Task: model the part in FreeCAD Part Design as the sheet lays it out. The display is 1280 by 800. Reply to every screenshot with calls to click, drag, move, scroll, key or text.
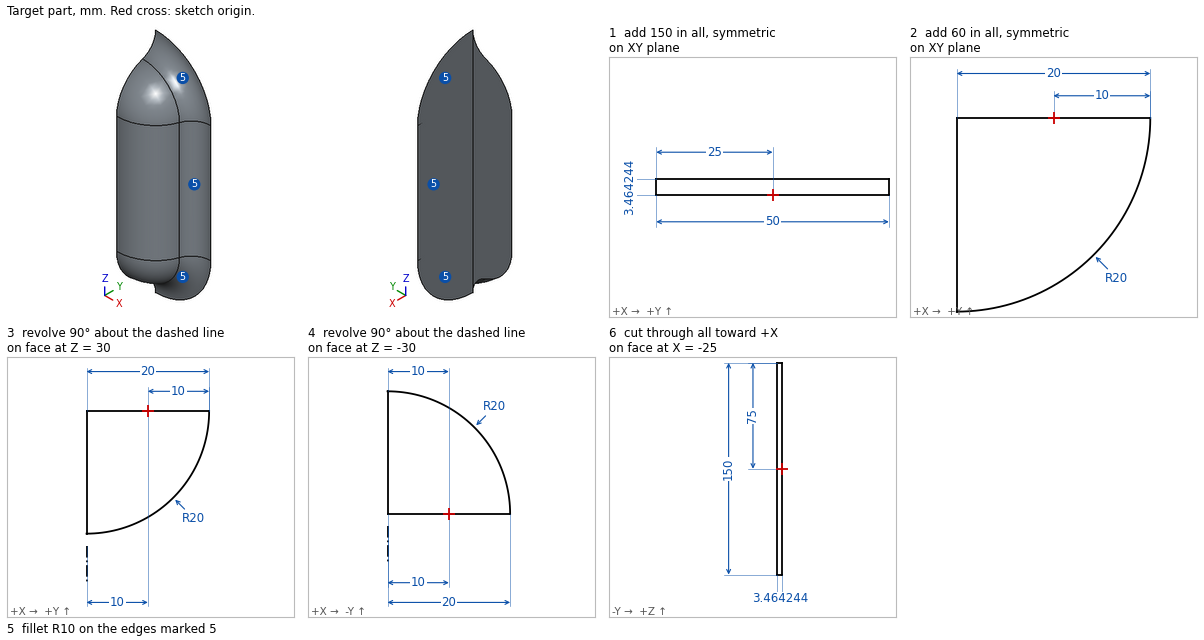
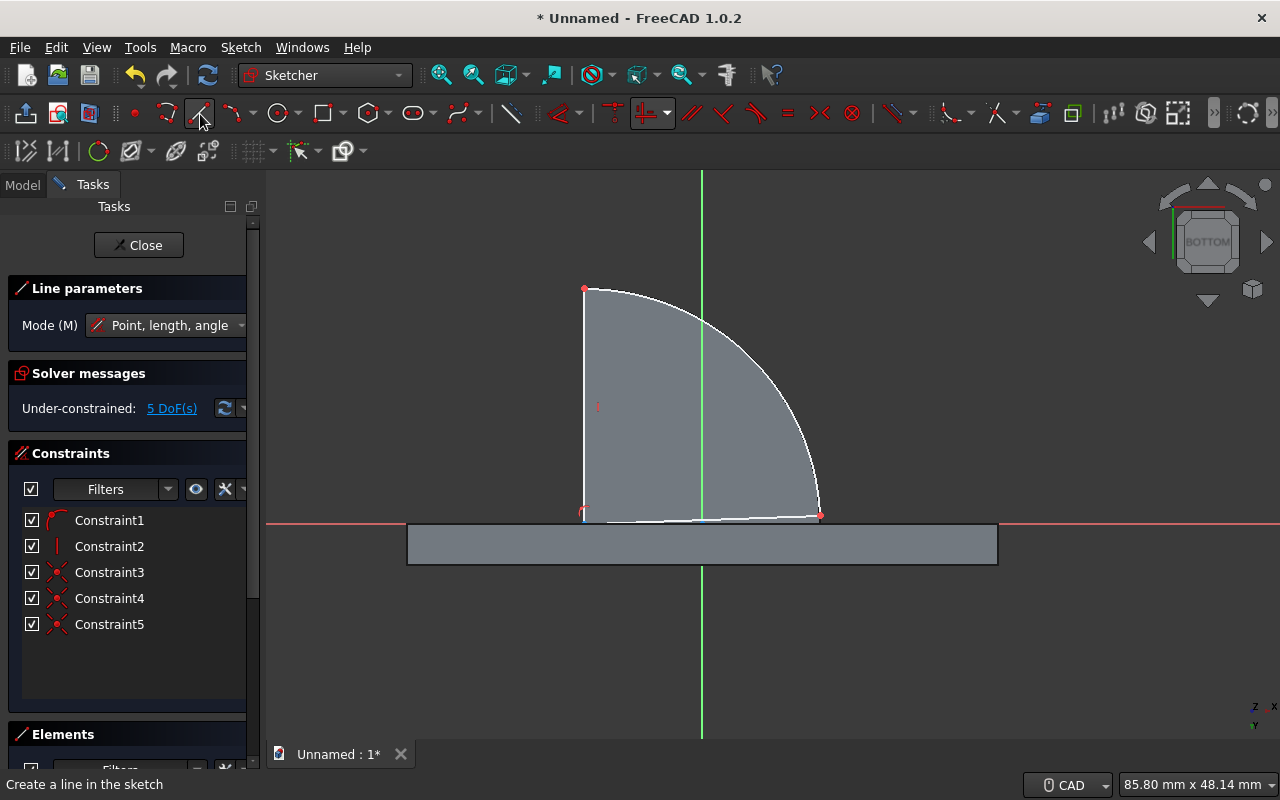
click(584, 548)
click(584, 619)
key(Escape)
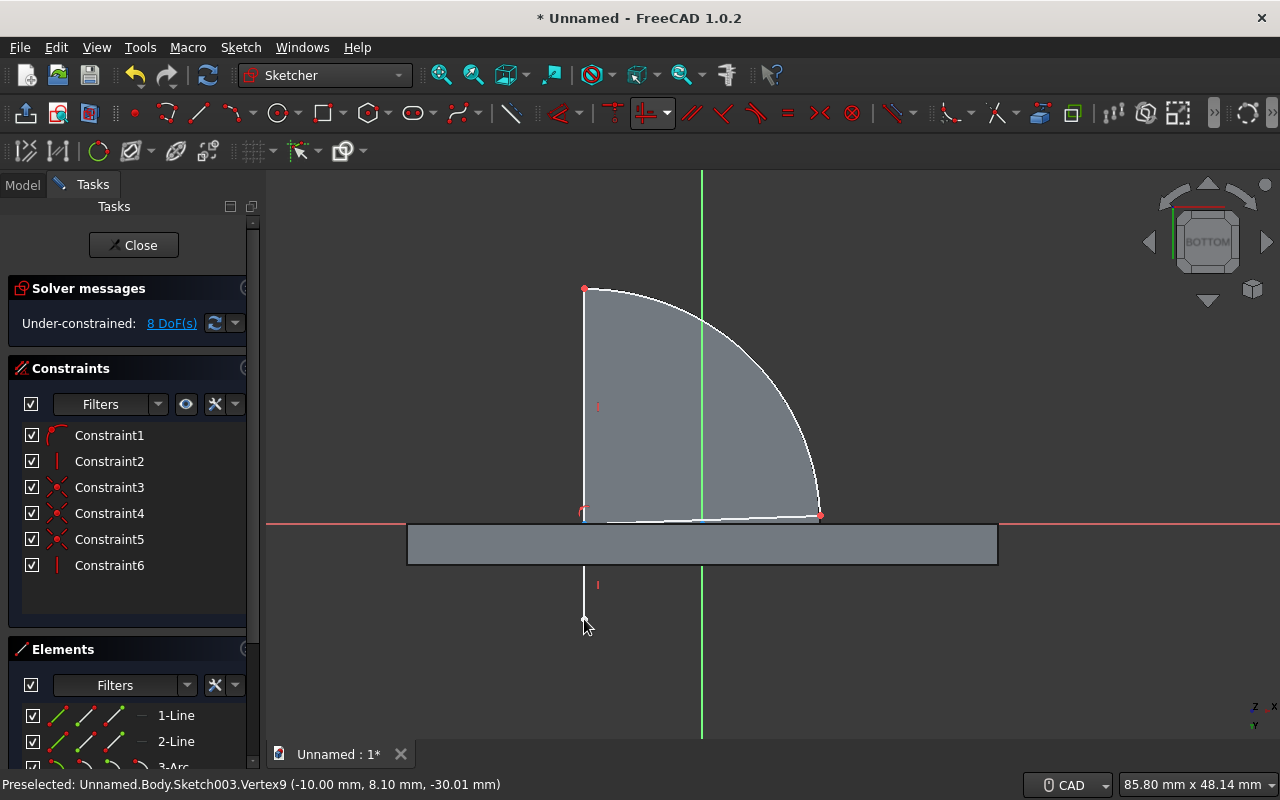
click(584, 570)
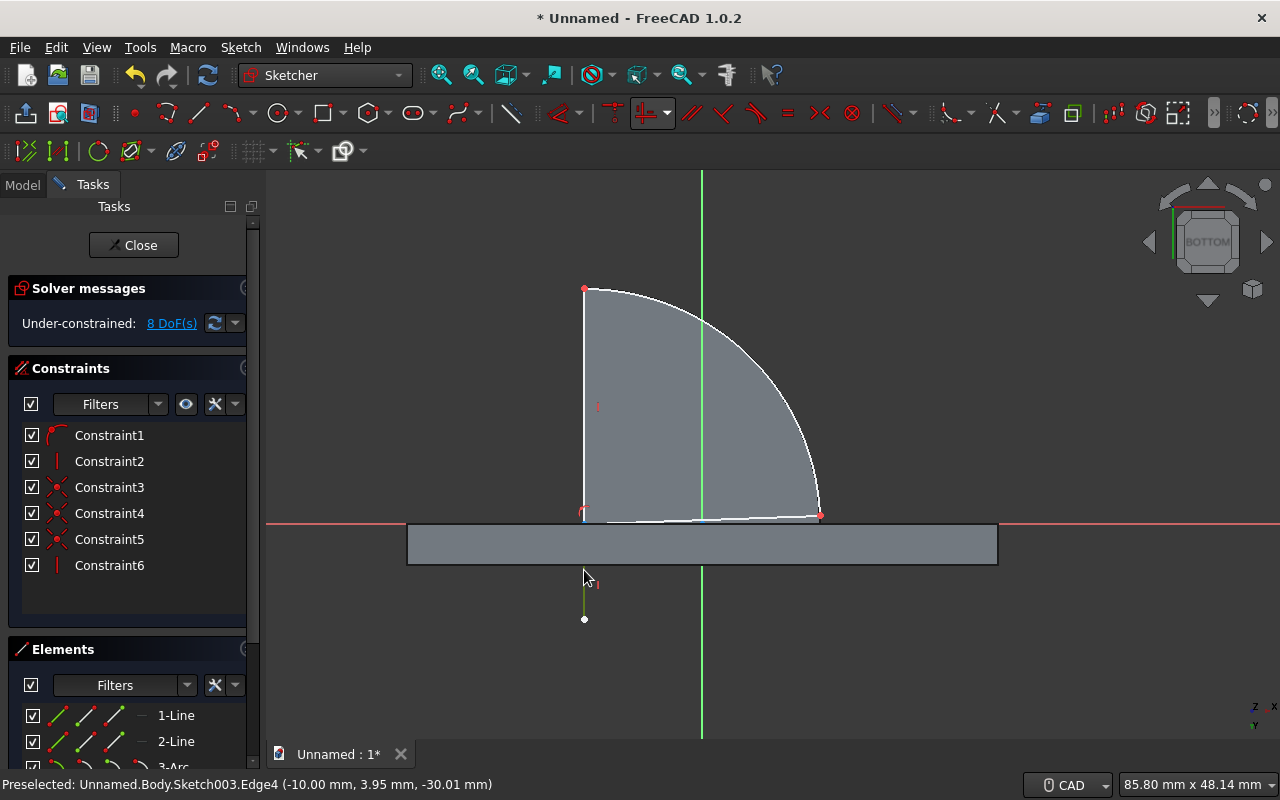
click(512, 114)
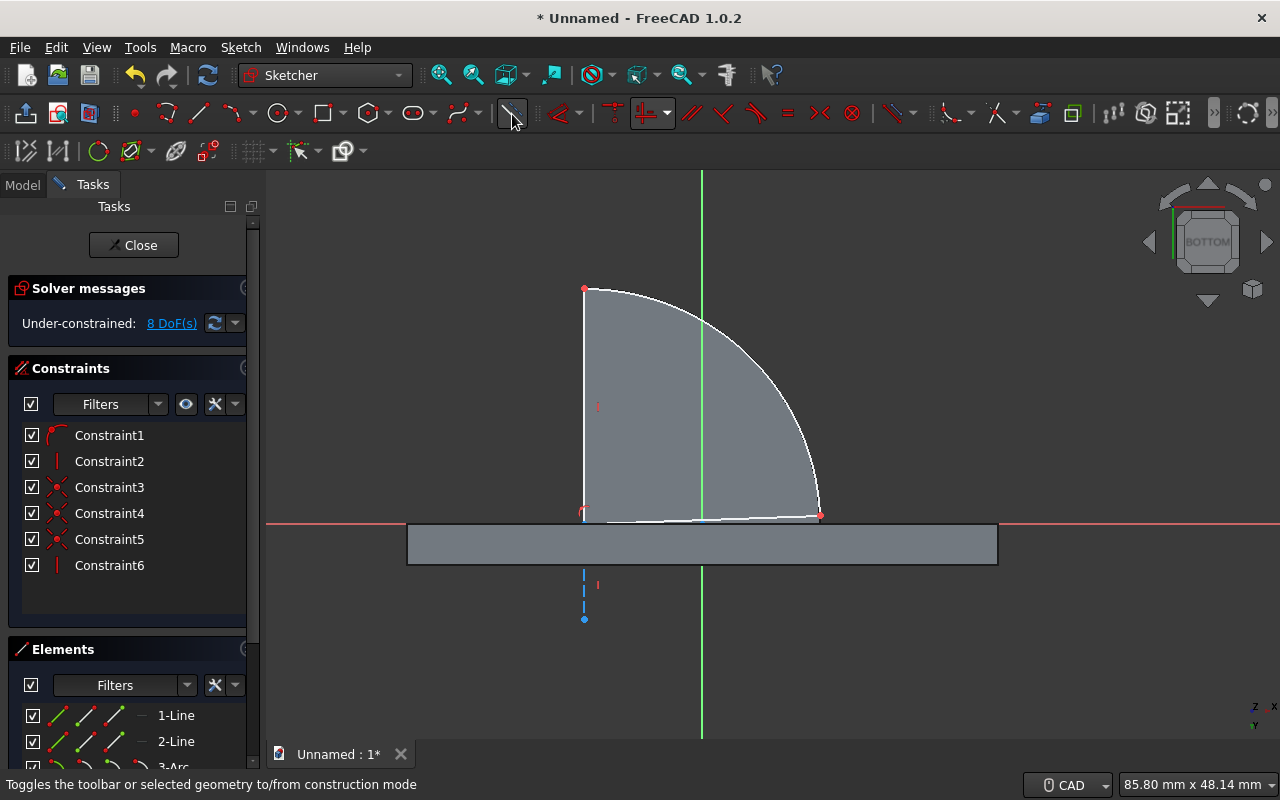
click(655, 522)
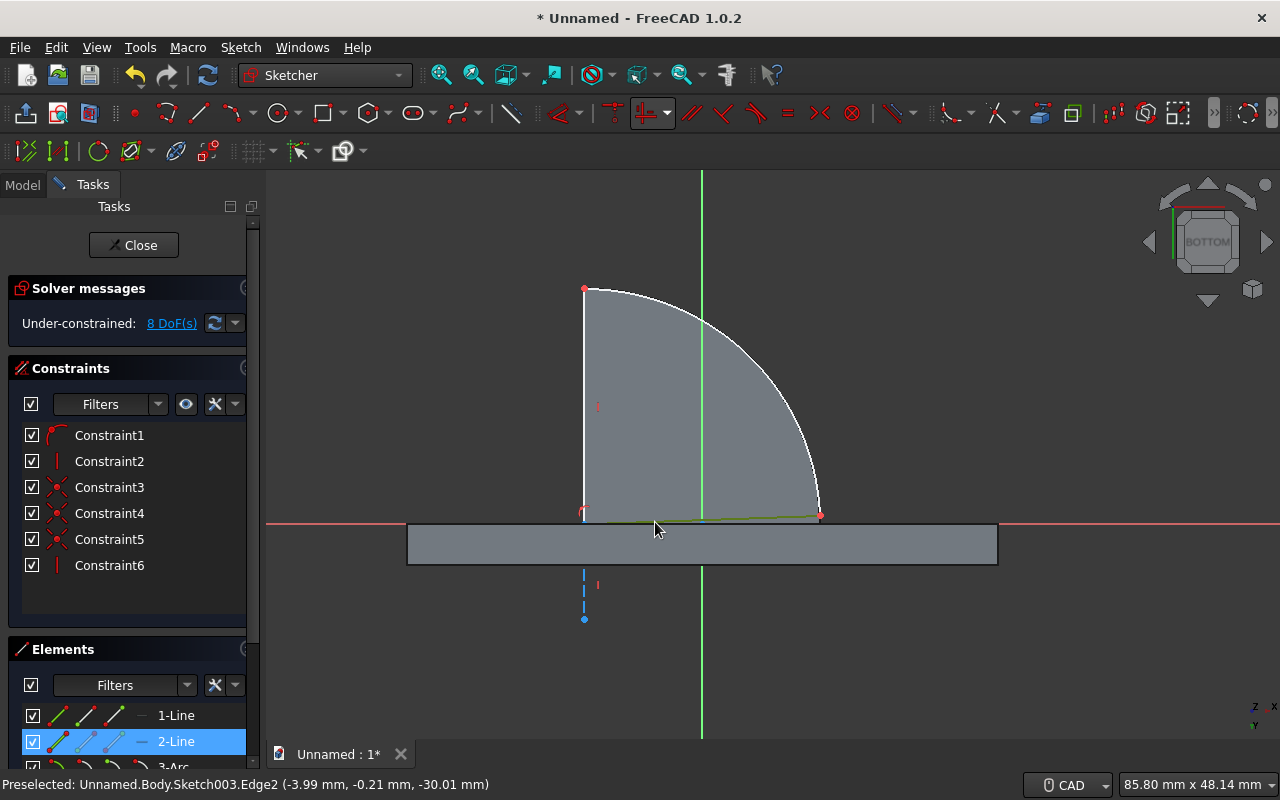
click(670, 114)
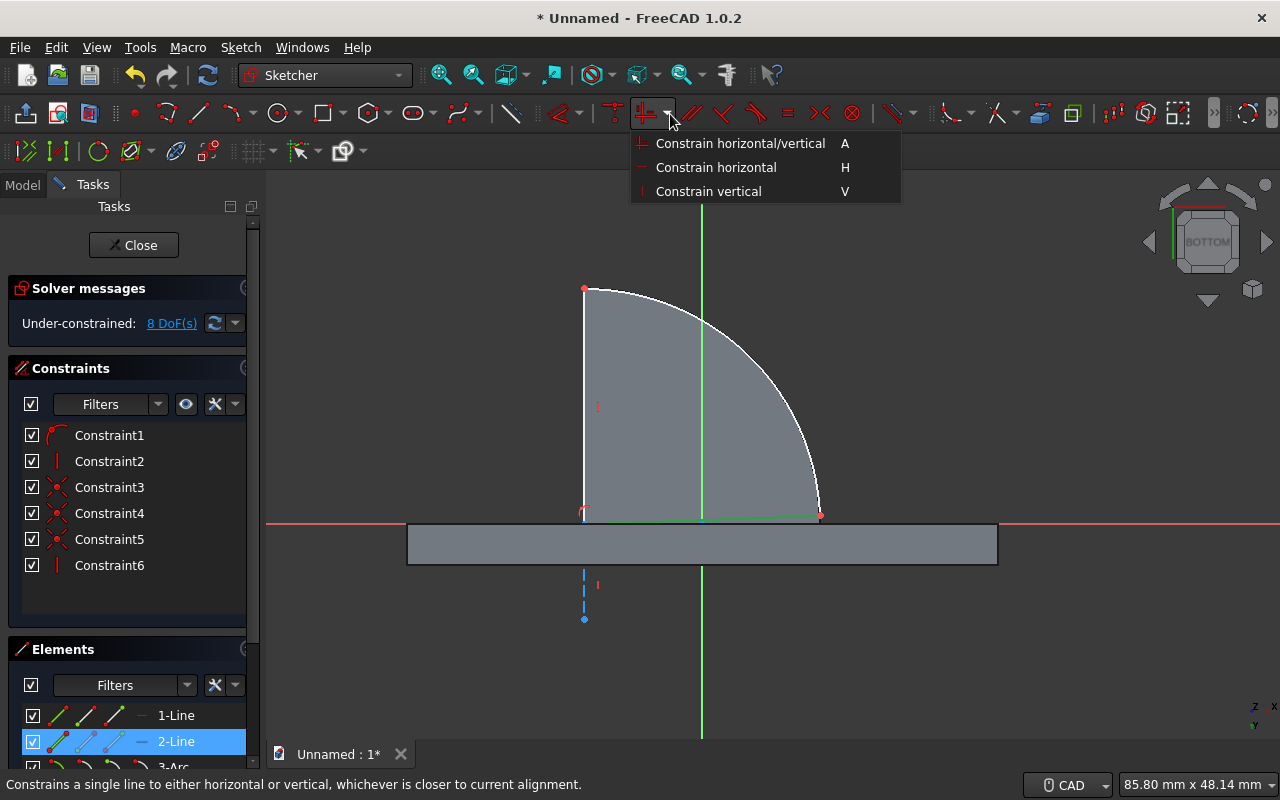
click(766, 167)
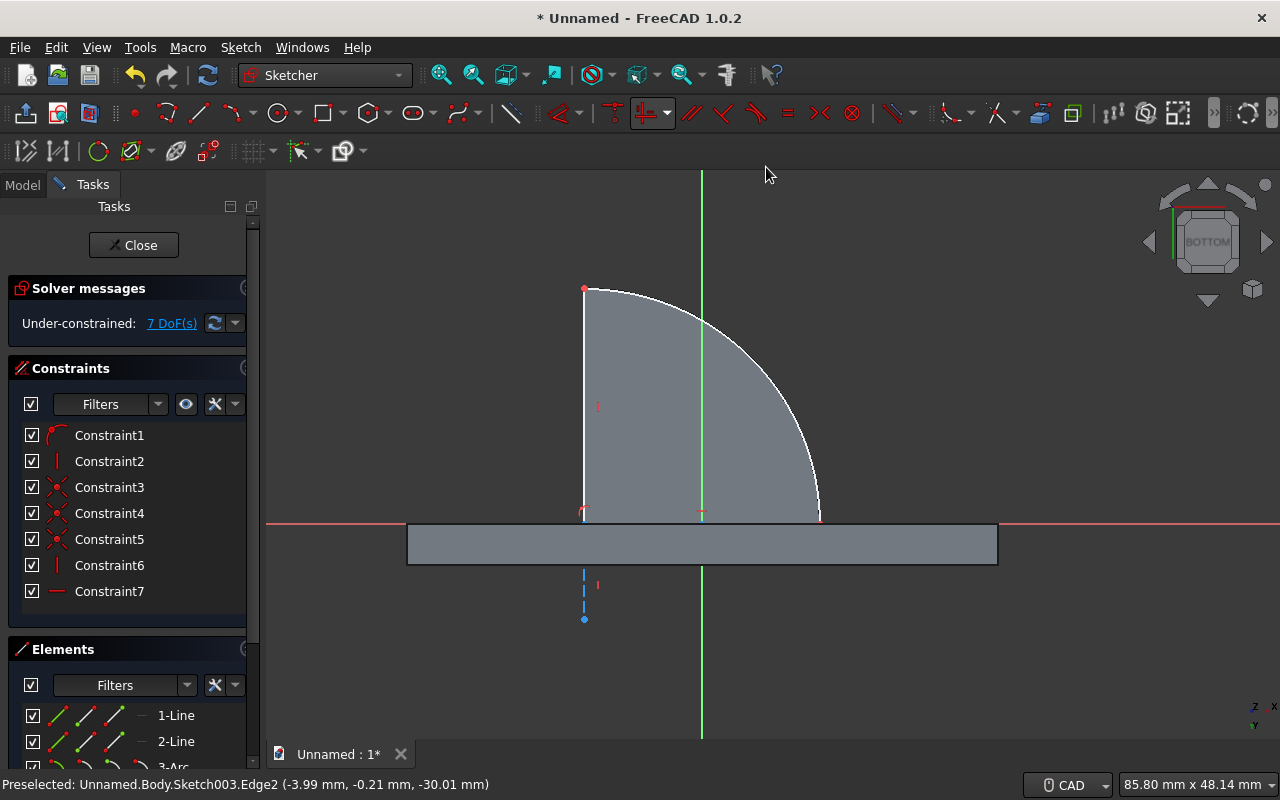
click(584, 525)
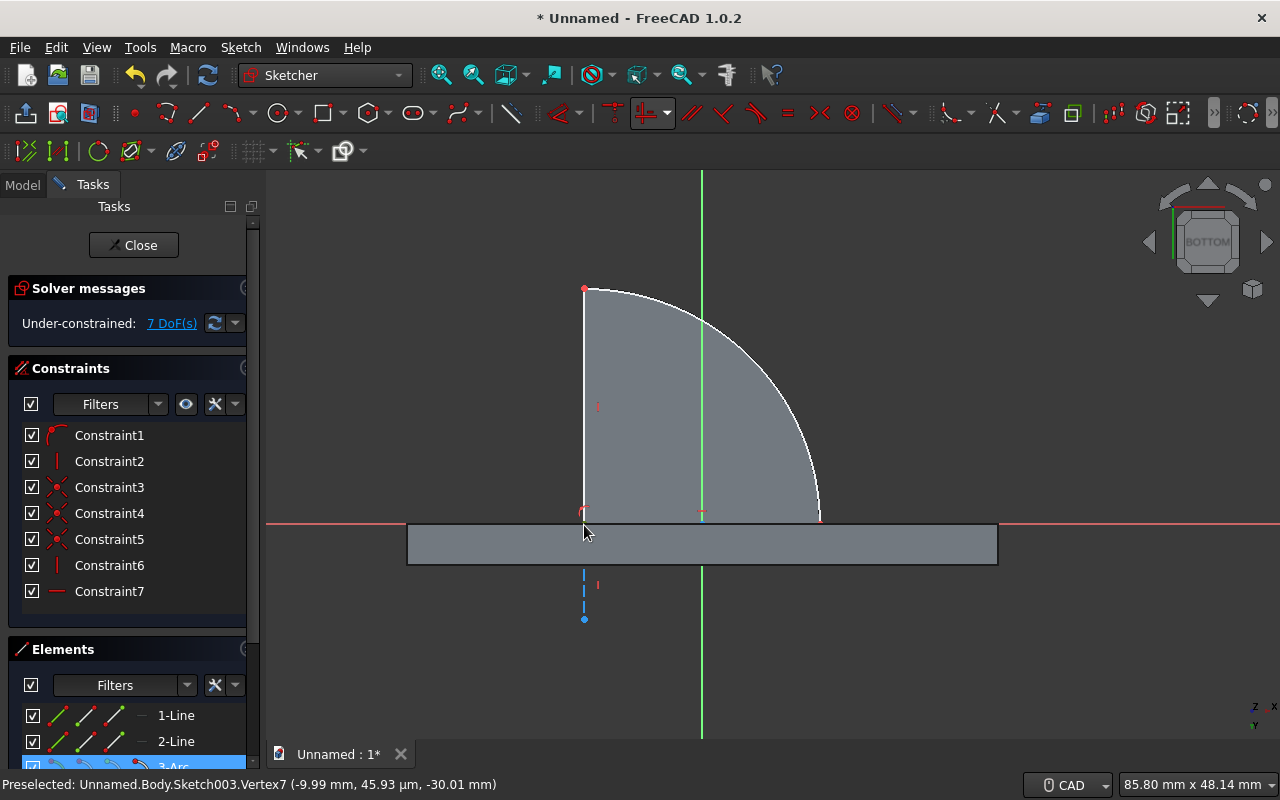
click(353, 524)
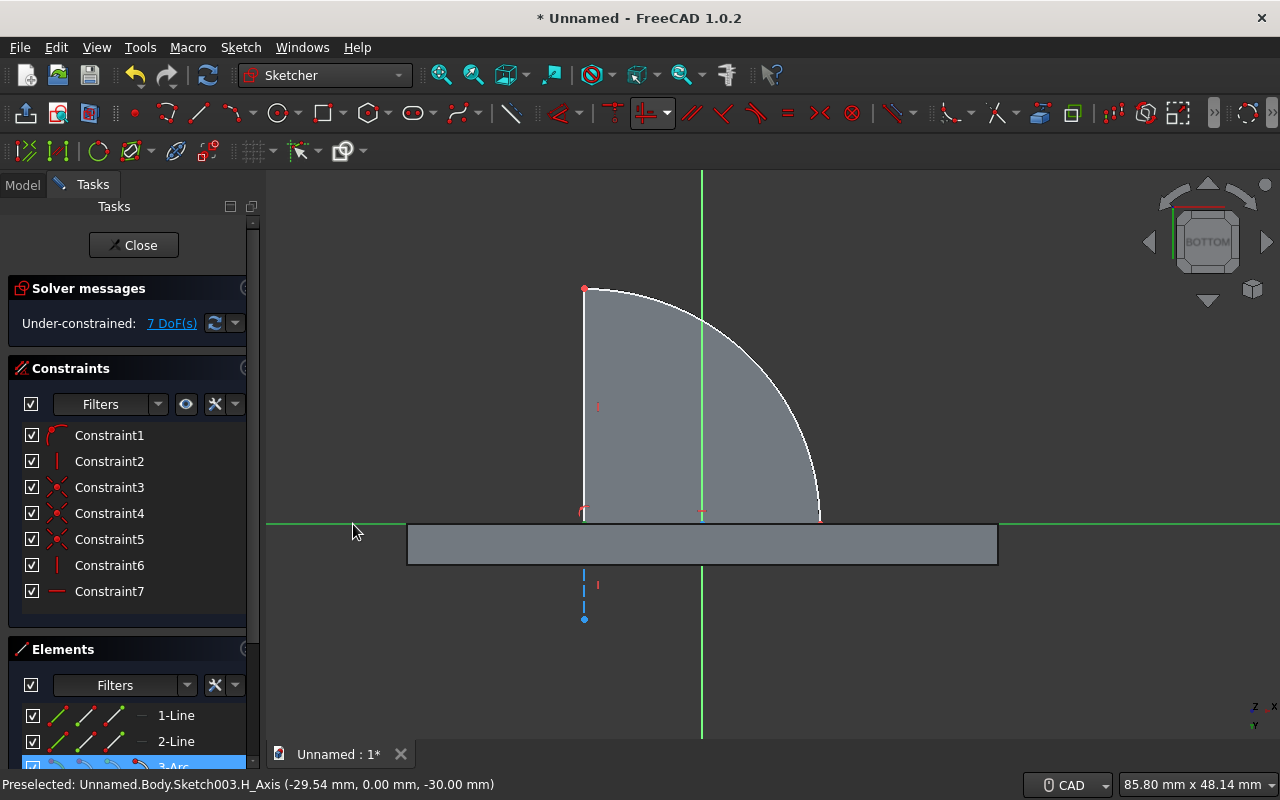
click(614, 114)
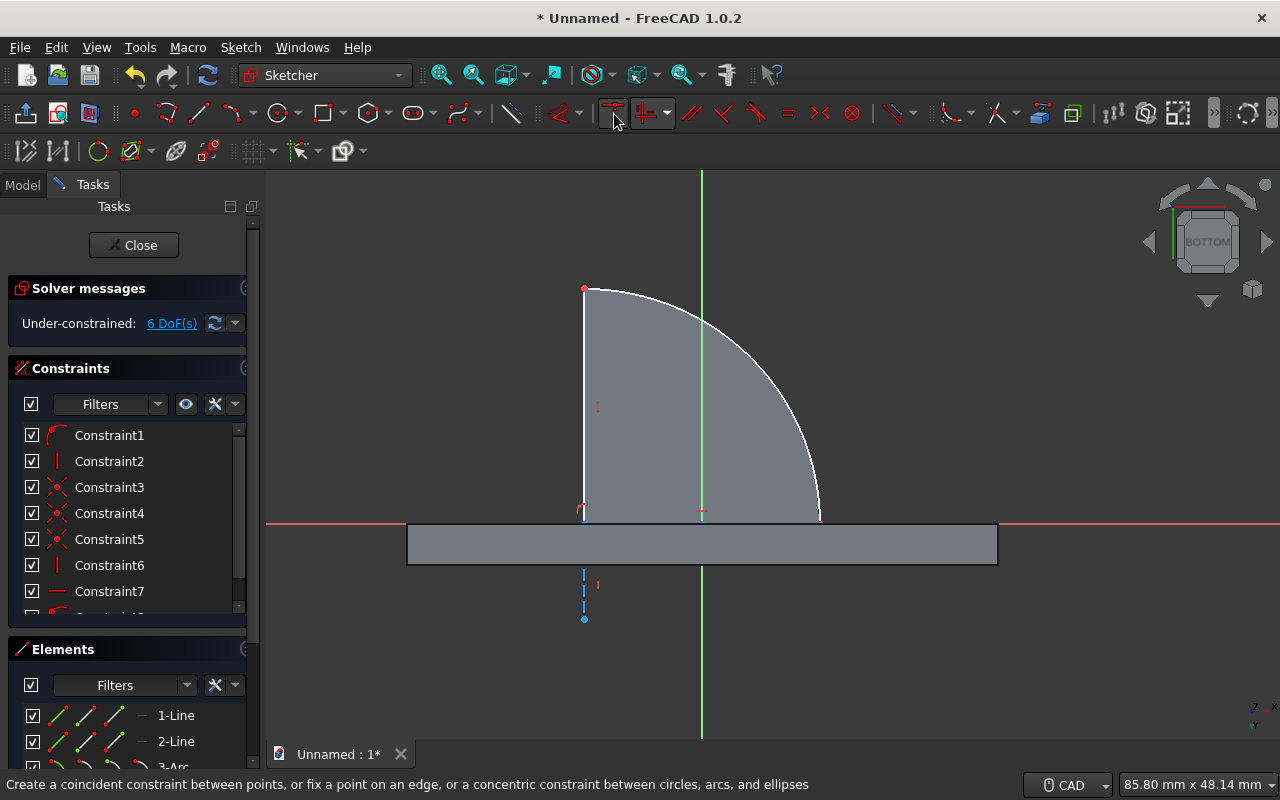
click(558, 114)